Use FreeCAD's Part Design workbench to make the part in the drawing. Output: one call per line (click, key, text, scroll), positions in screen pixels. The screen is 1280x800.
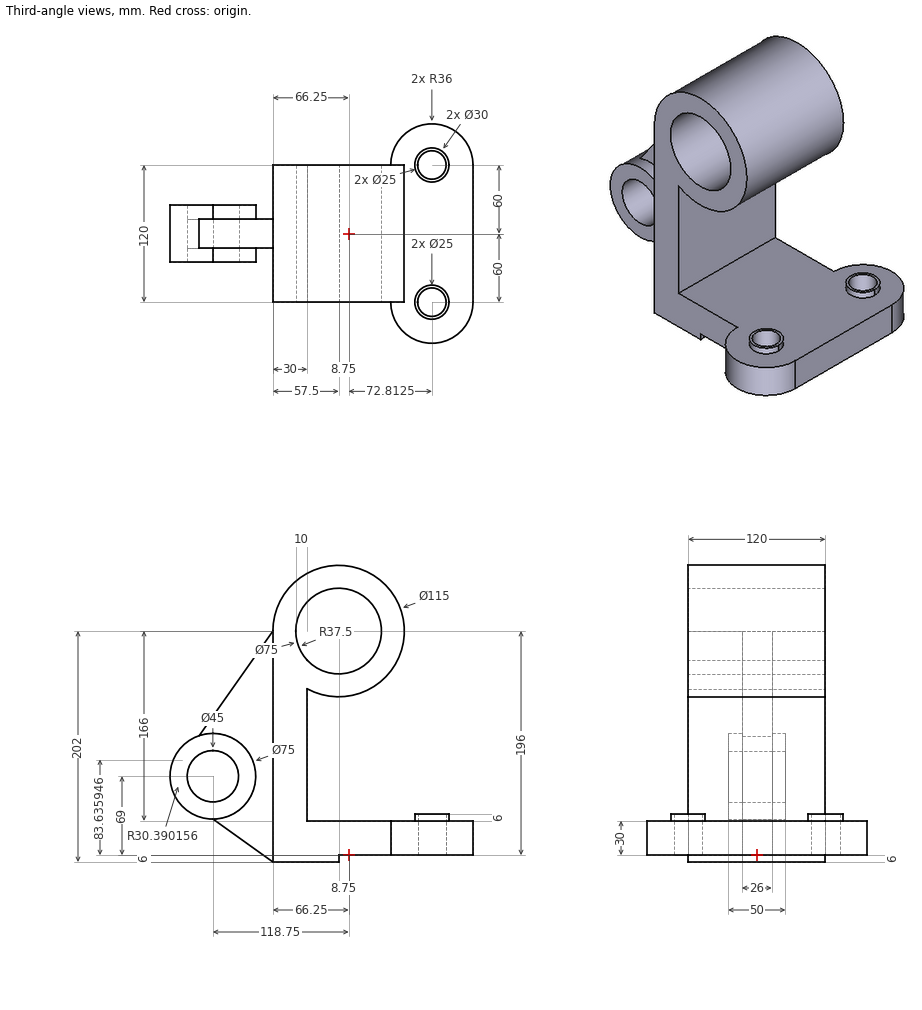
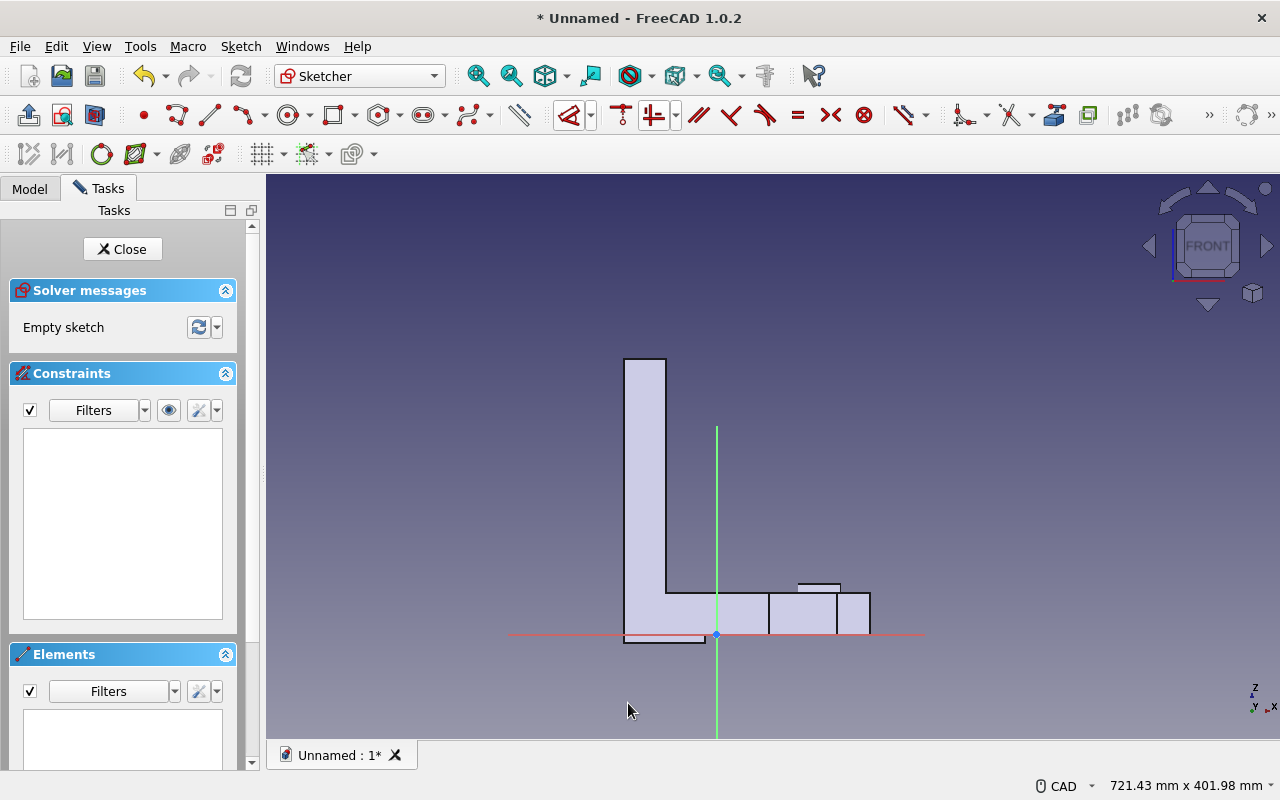
key(g)
key(c)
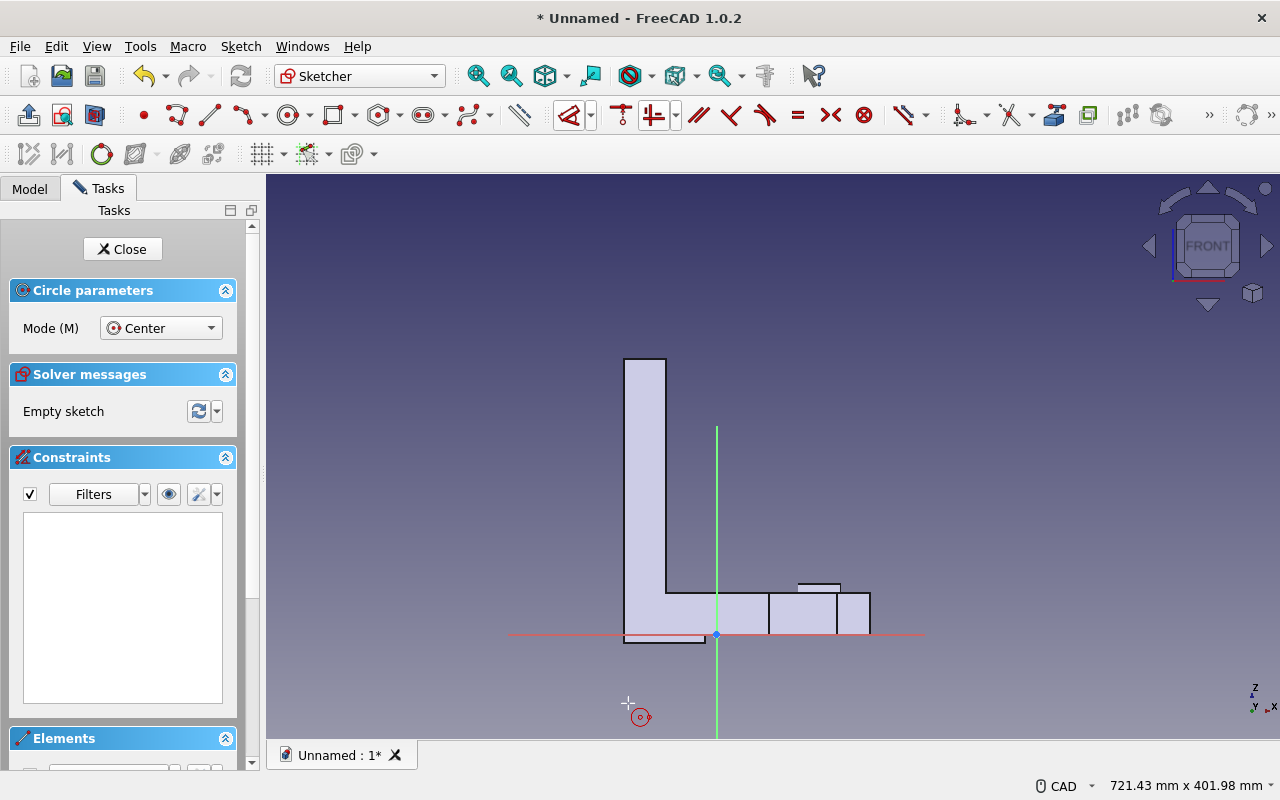
scroll(705, 359, up, 2)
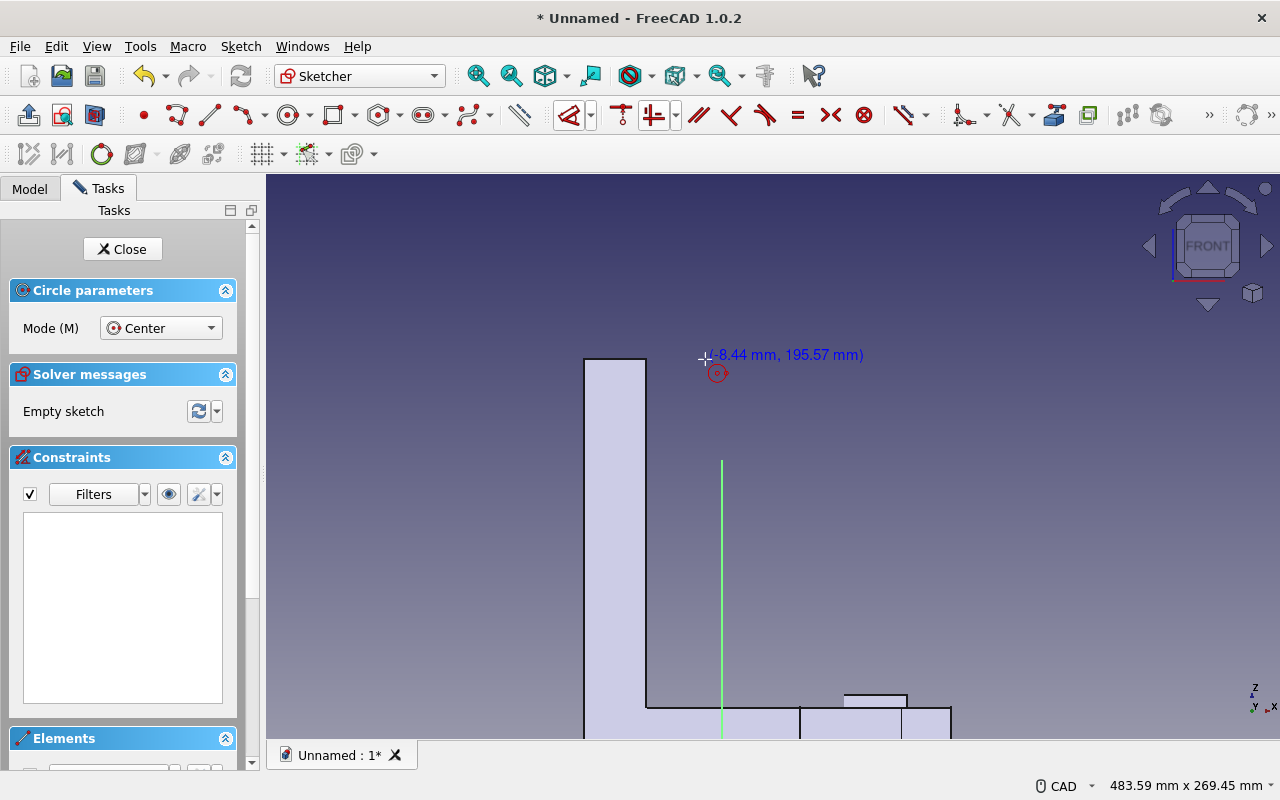
click(704, 359)
click(789, 274)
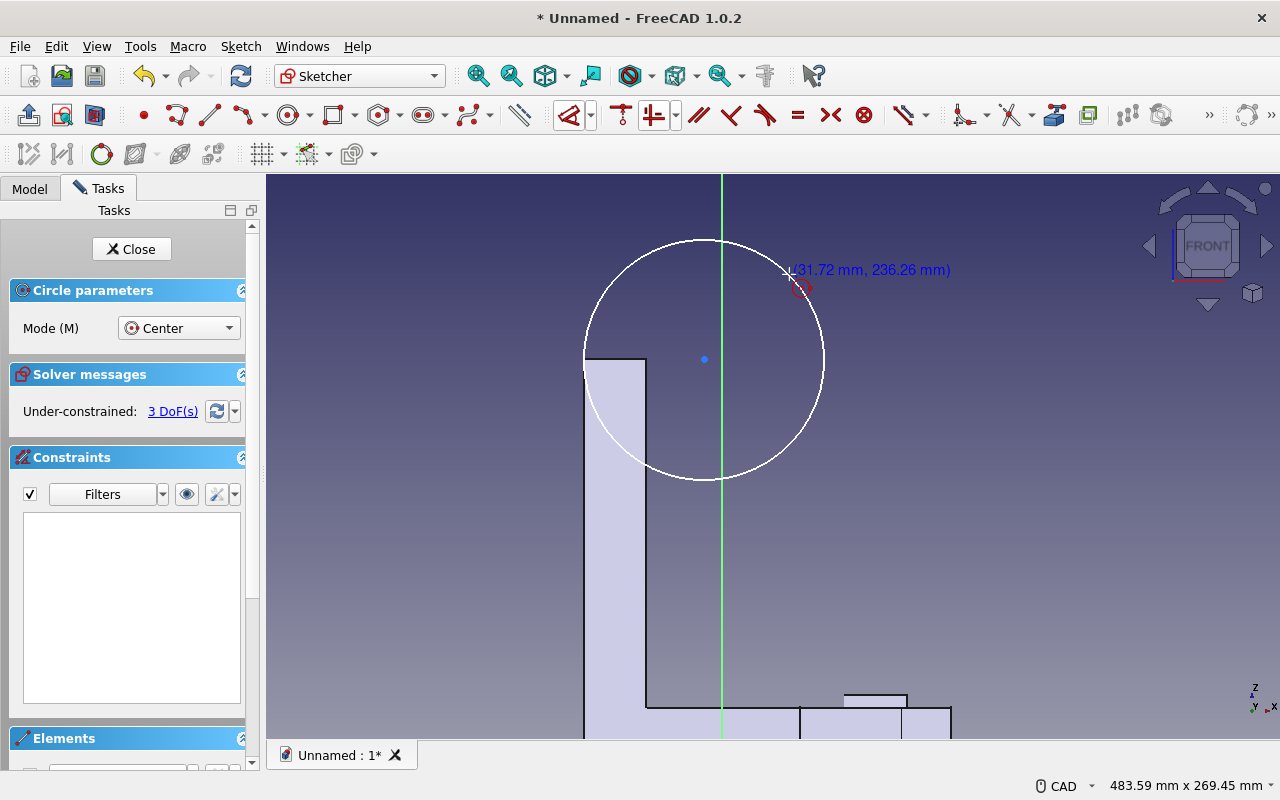
click(704, 360)
click(760, 304)
key(Escape)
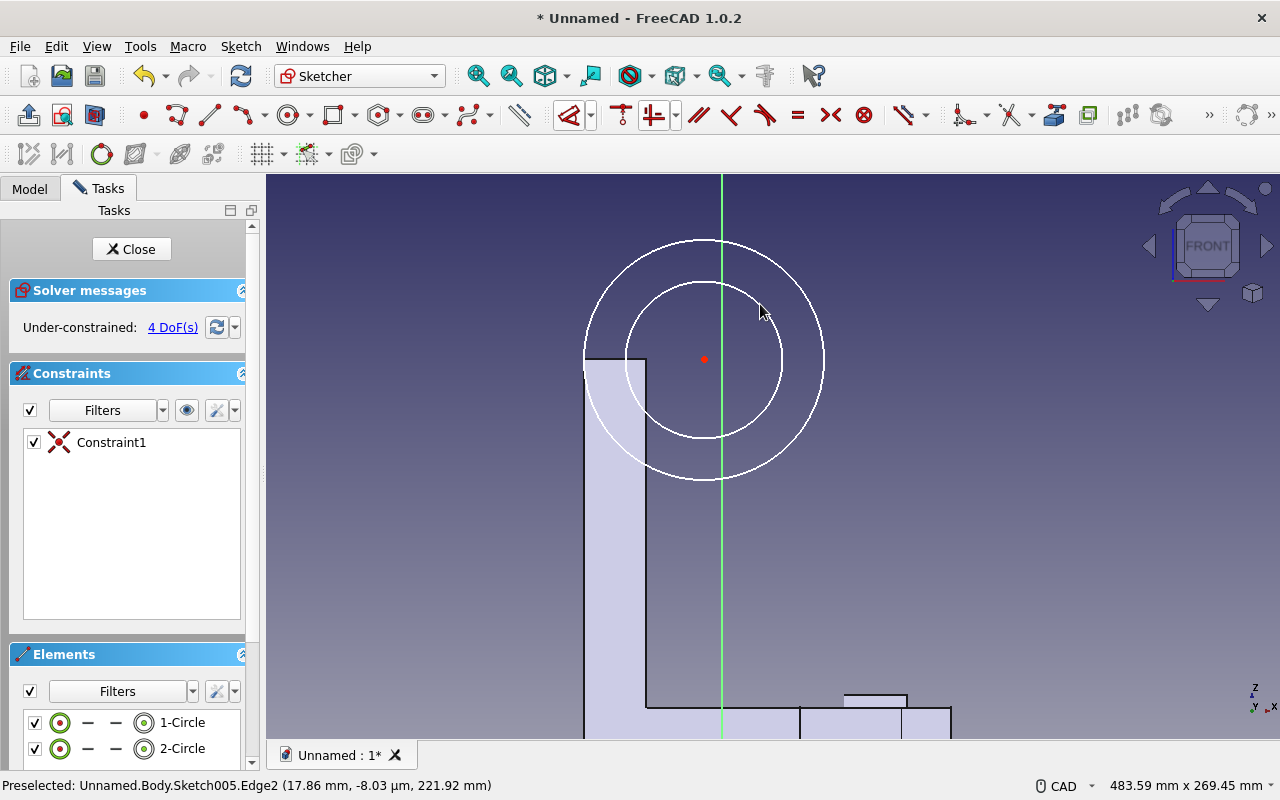
click(789, 275)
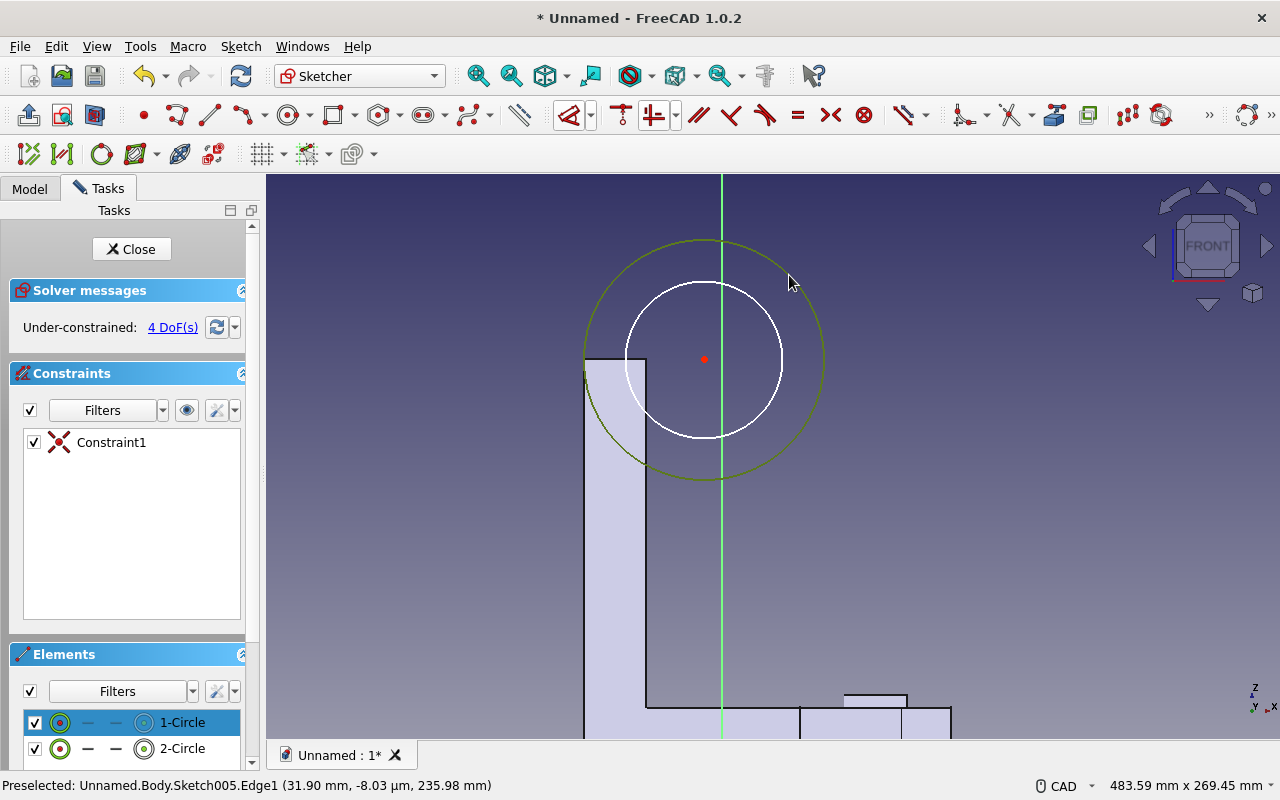
key(k)
key(o)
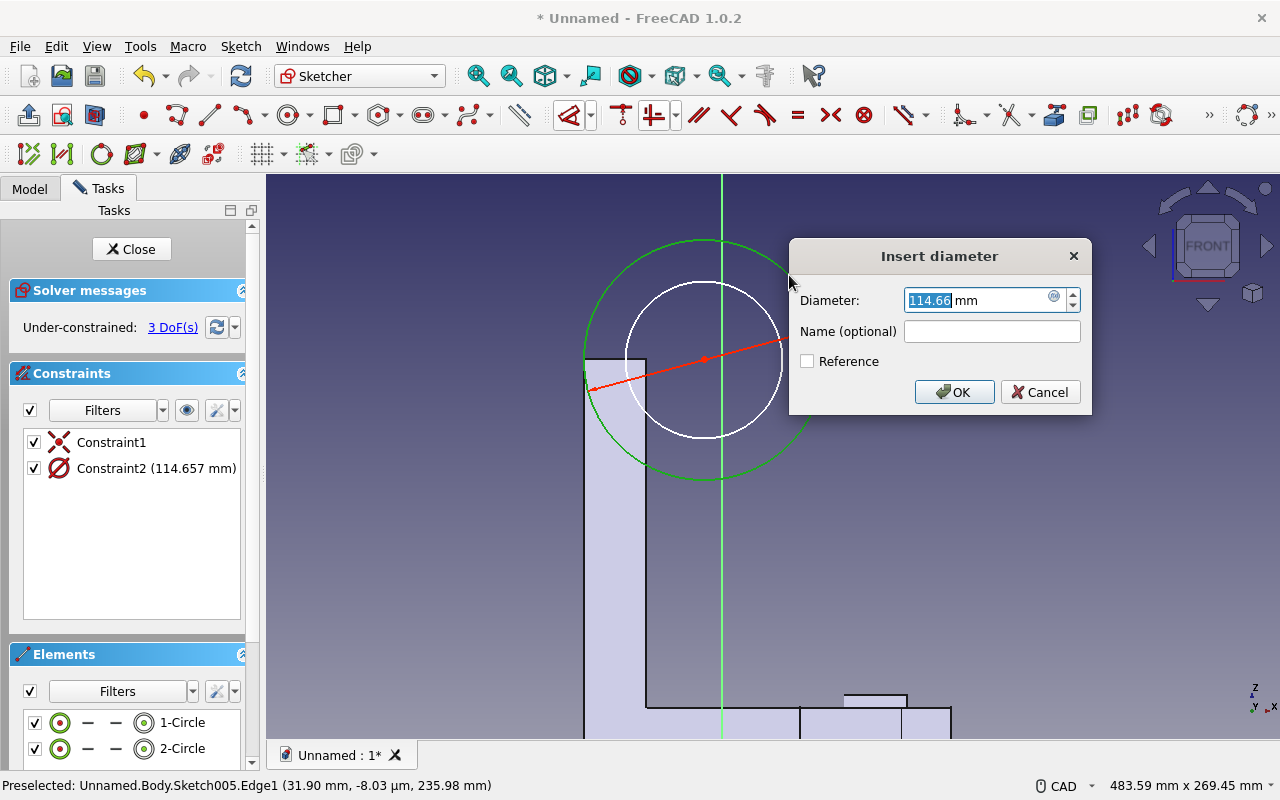
text(115)
key(Return)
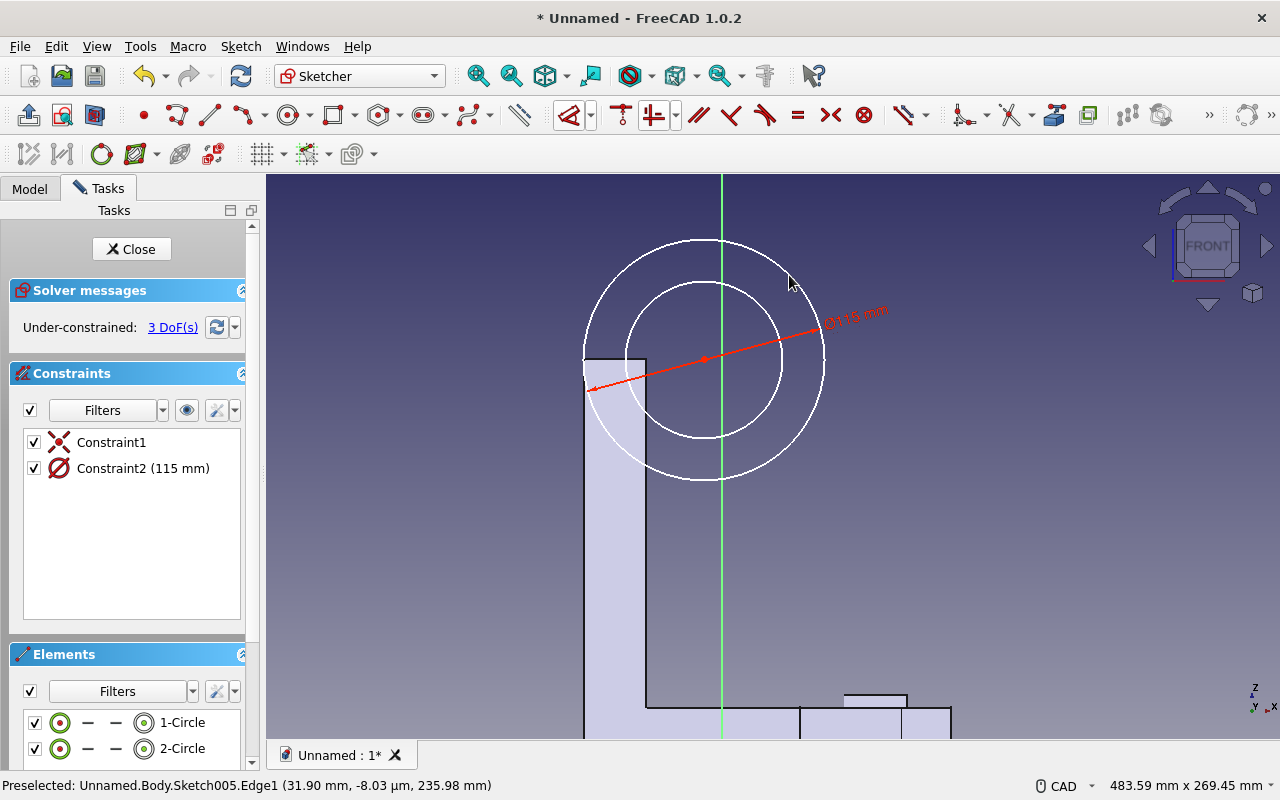
click(759, 304)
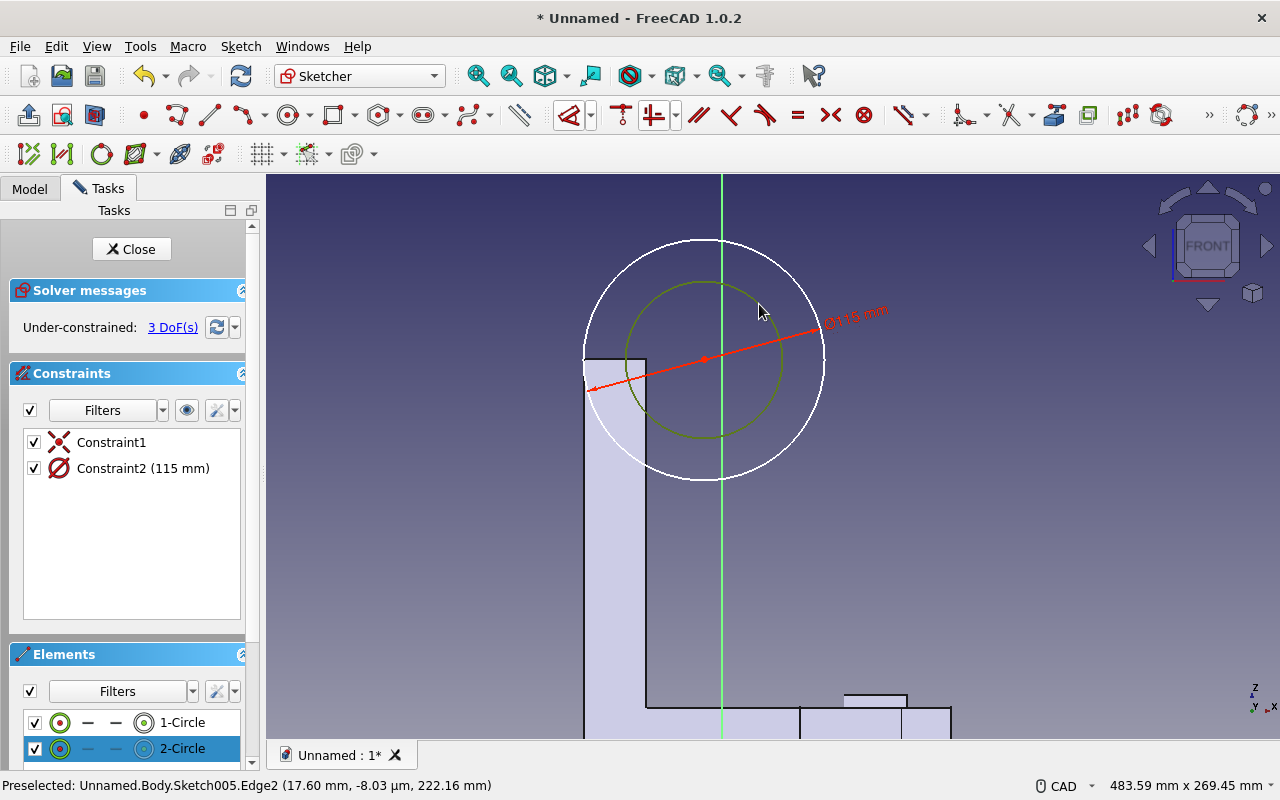
click(590, 116)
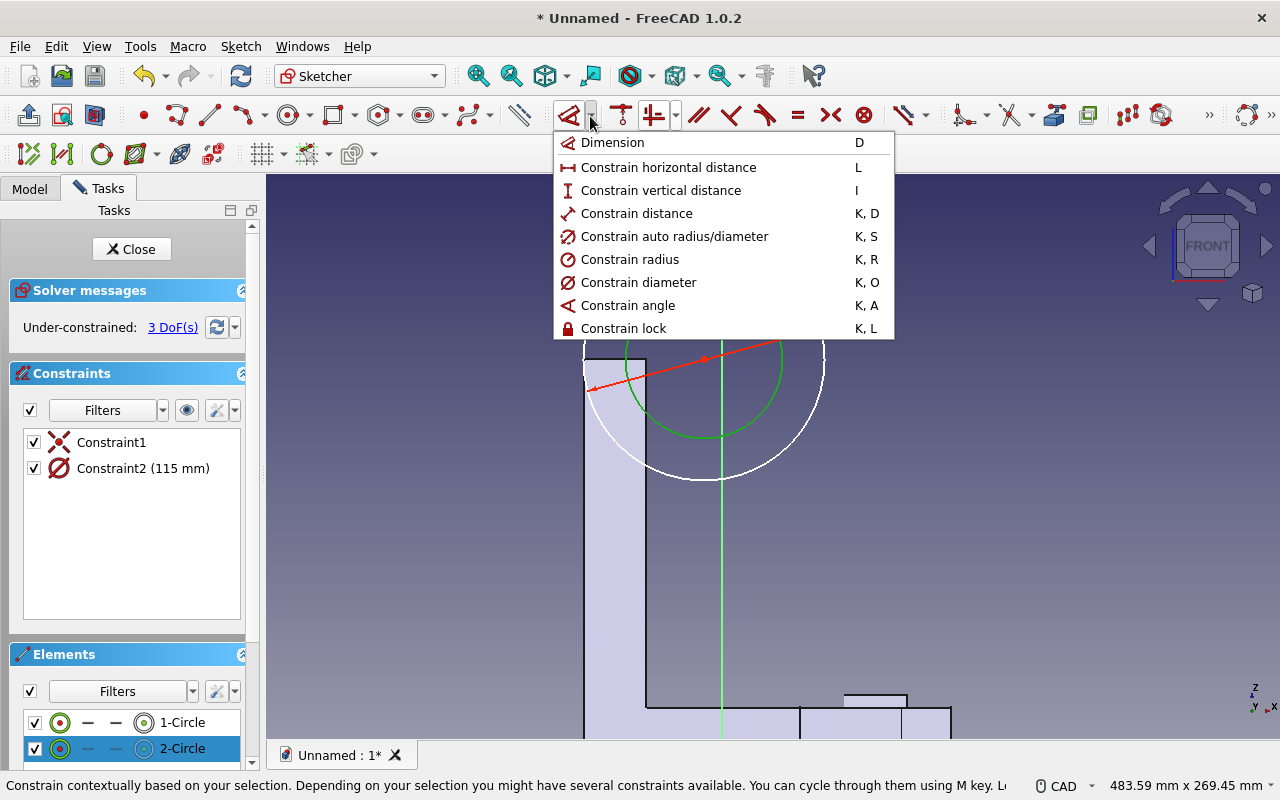
click(724, 282)